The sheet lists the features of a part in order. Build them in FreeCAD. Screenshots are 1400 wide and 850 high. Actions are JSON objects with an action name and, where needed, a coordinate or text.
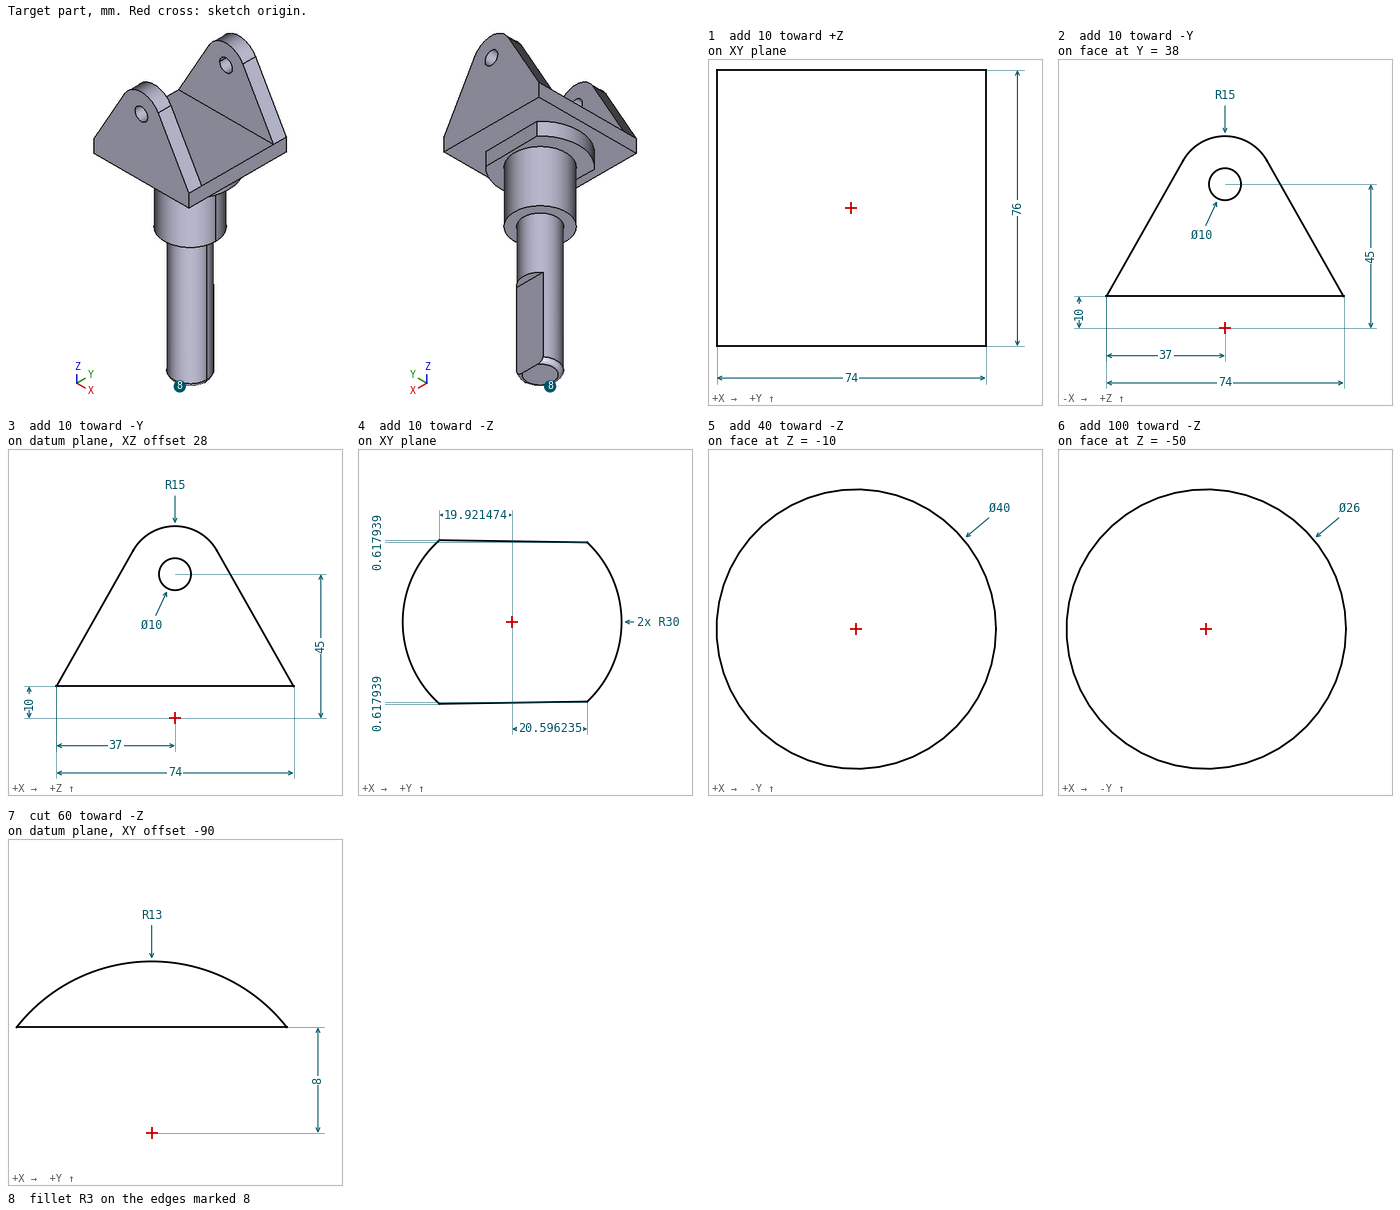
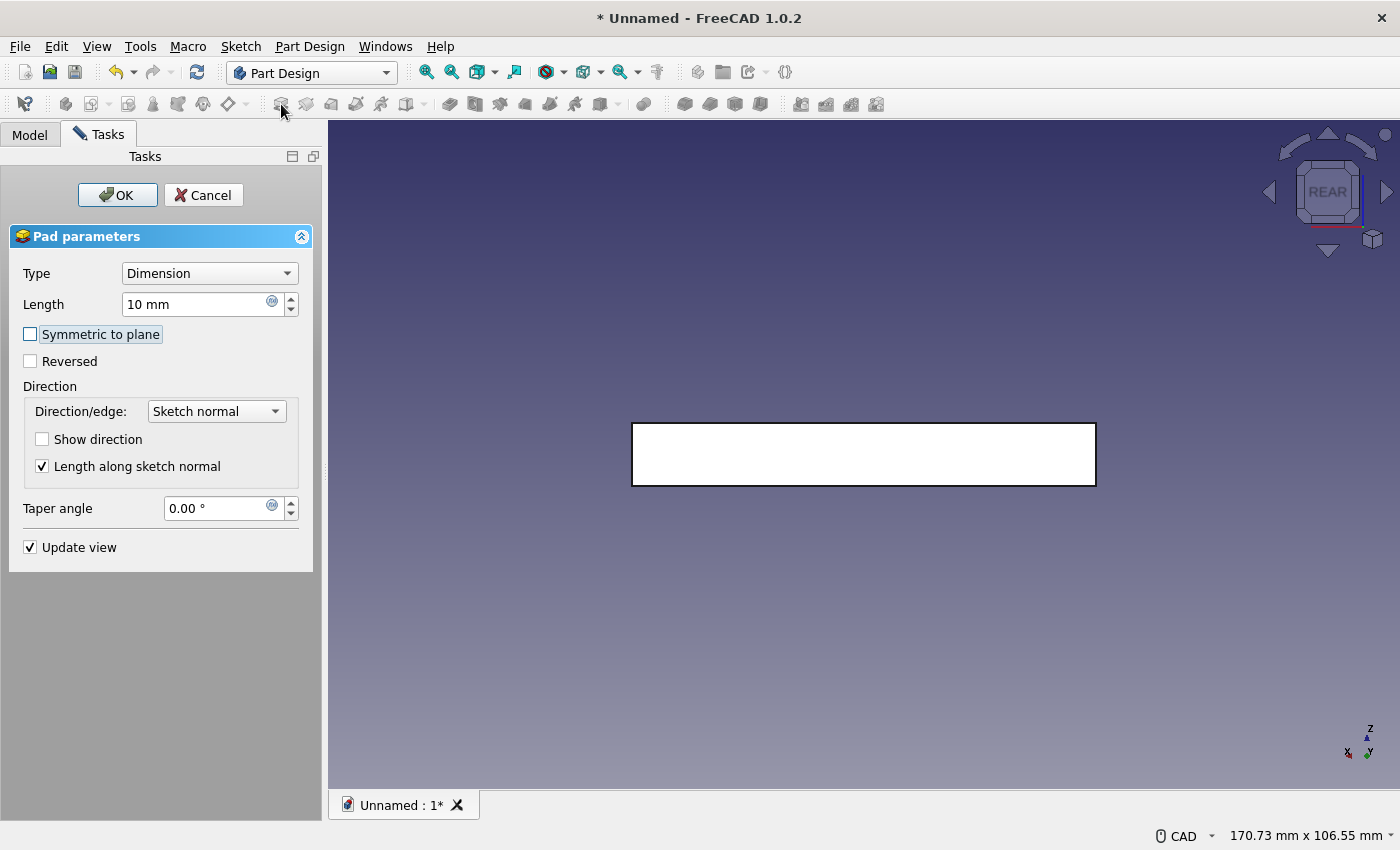
{"action": "left_click", "coordinate": [31, 361]}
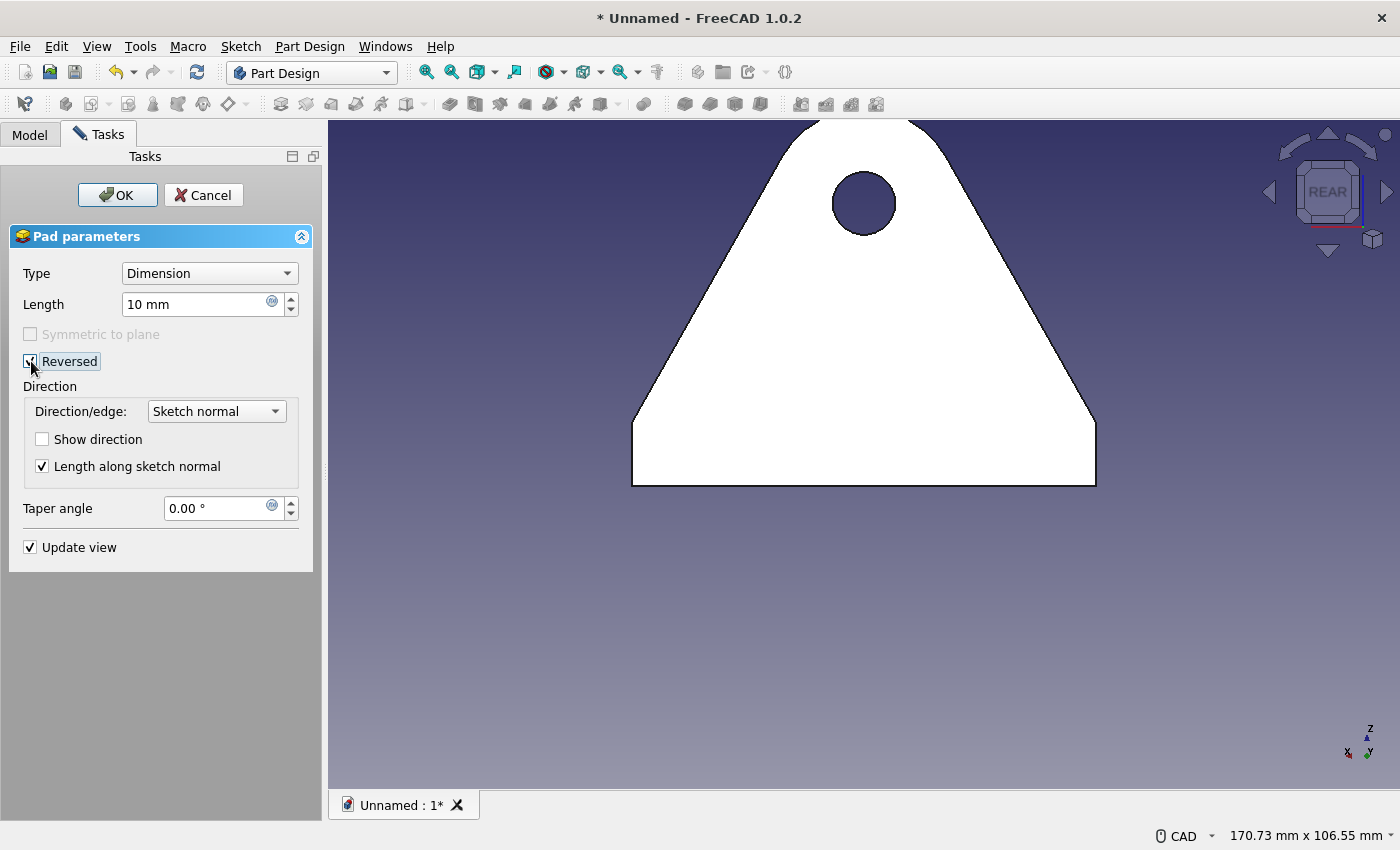
{"action": "left_click", "coordinate": [118, 195]}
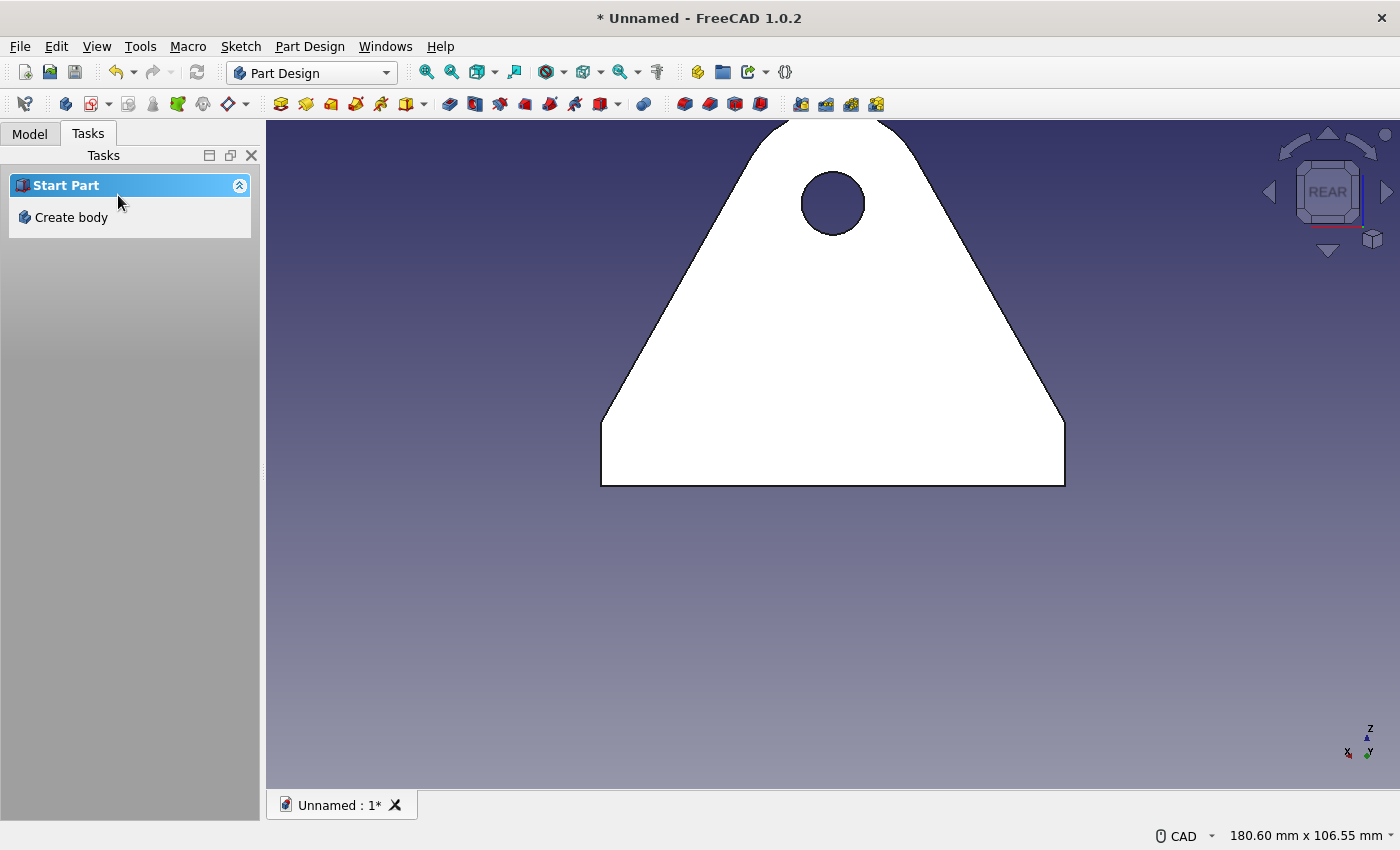
{"action": "left_click", "coordinate": [427, 72]}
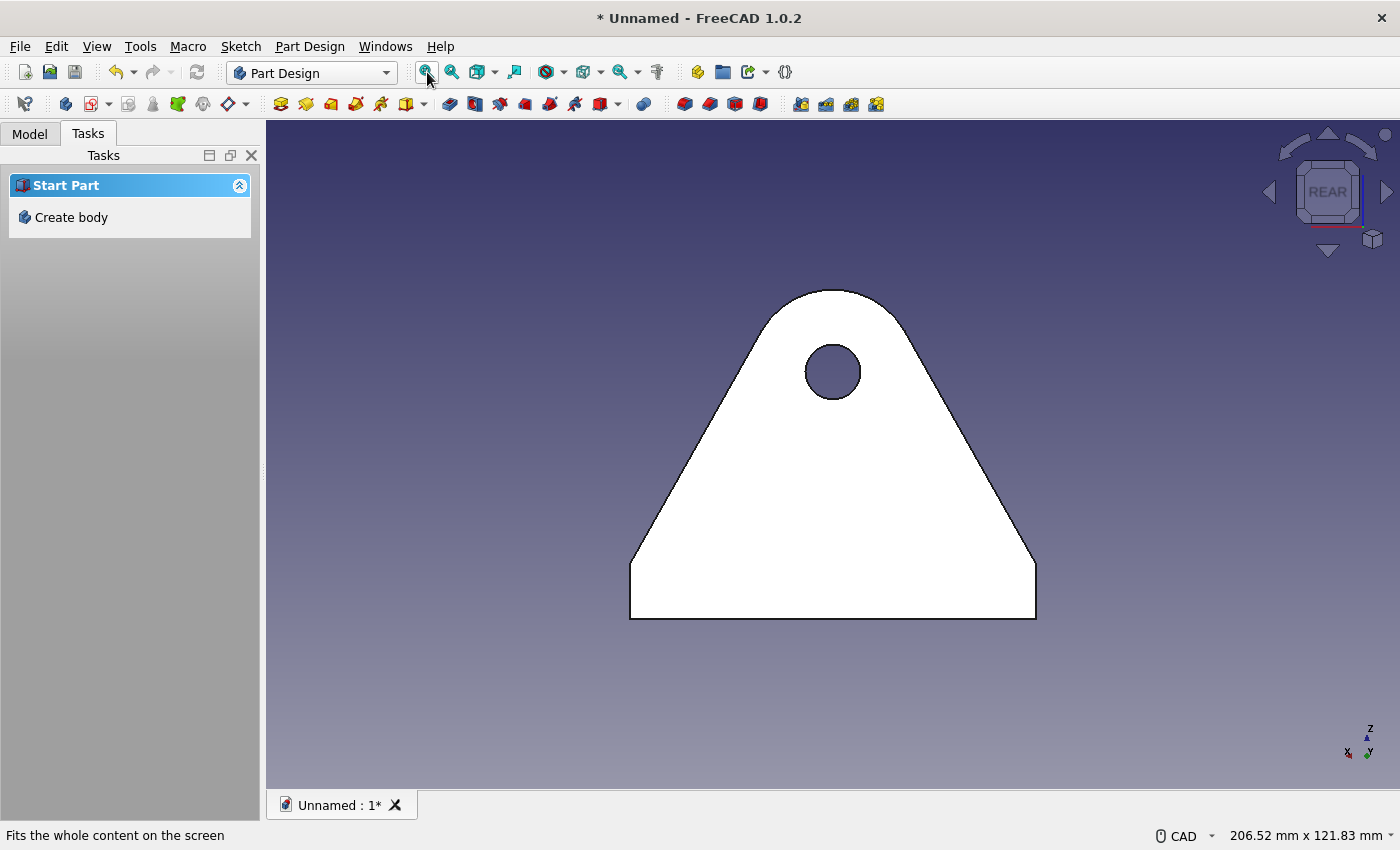
{"action": "left_click", "coordinate": [30, 134]}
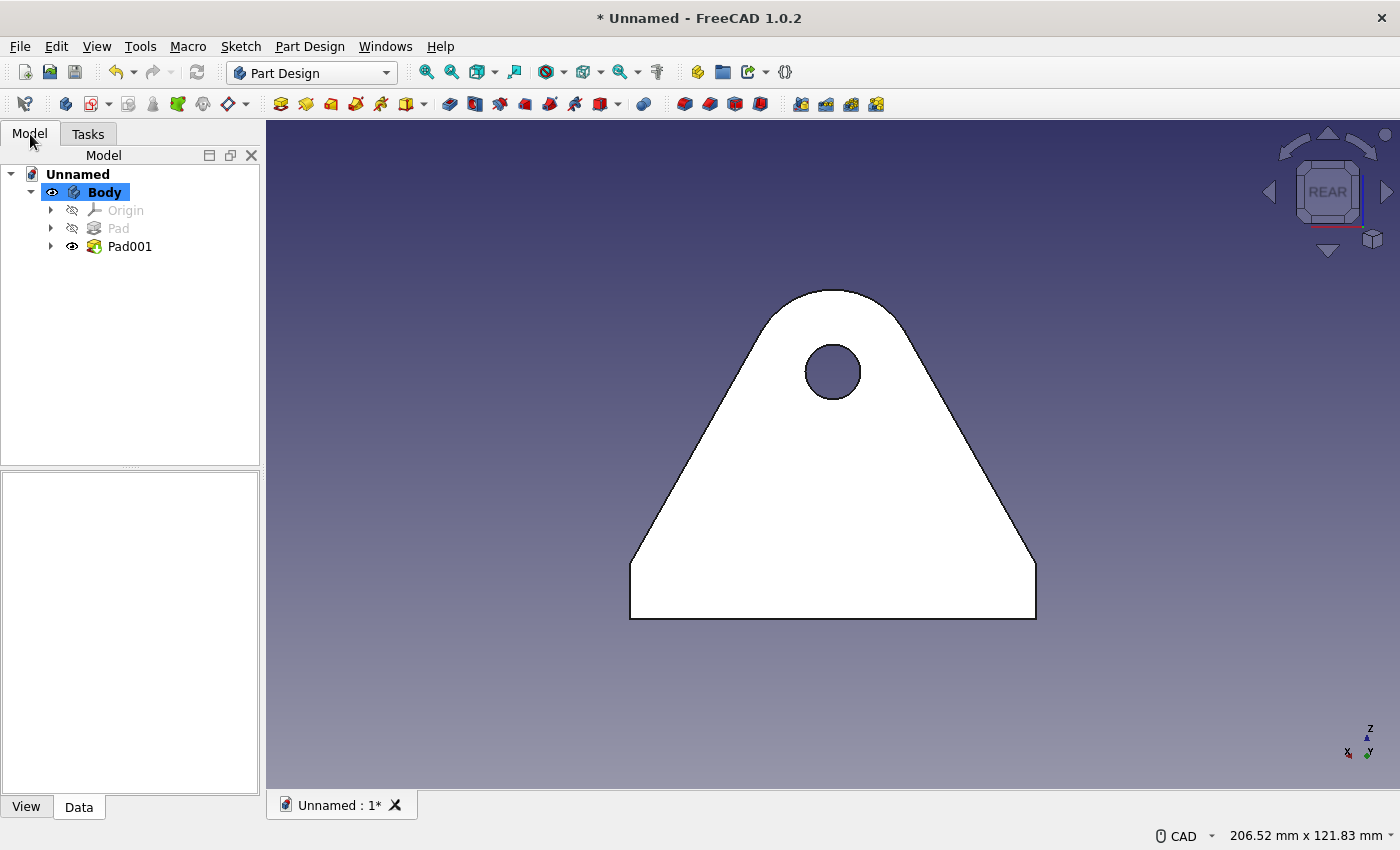
{"action": "left_click", "coordinate": [51, 210]}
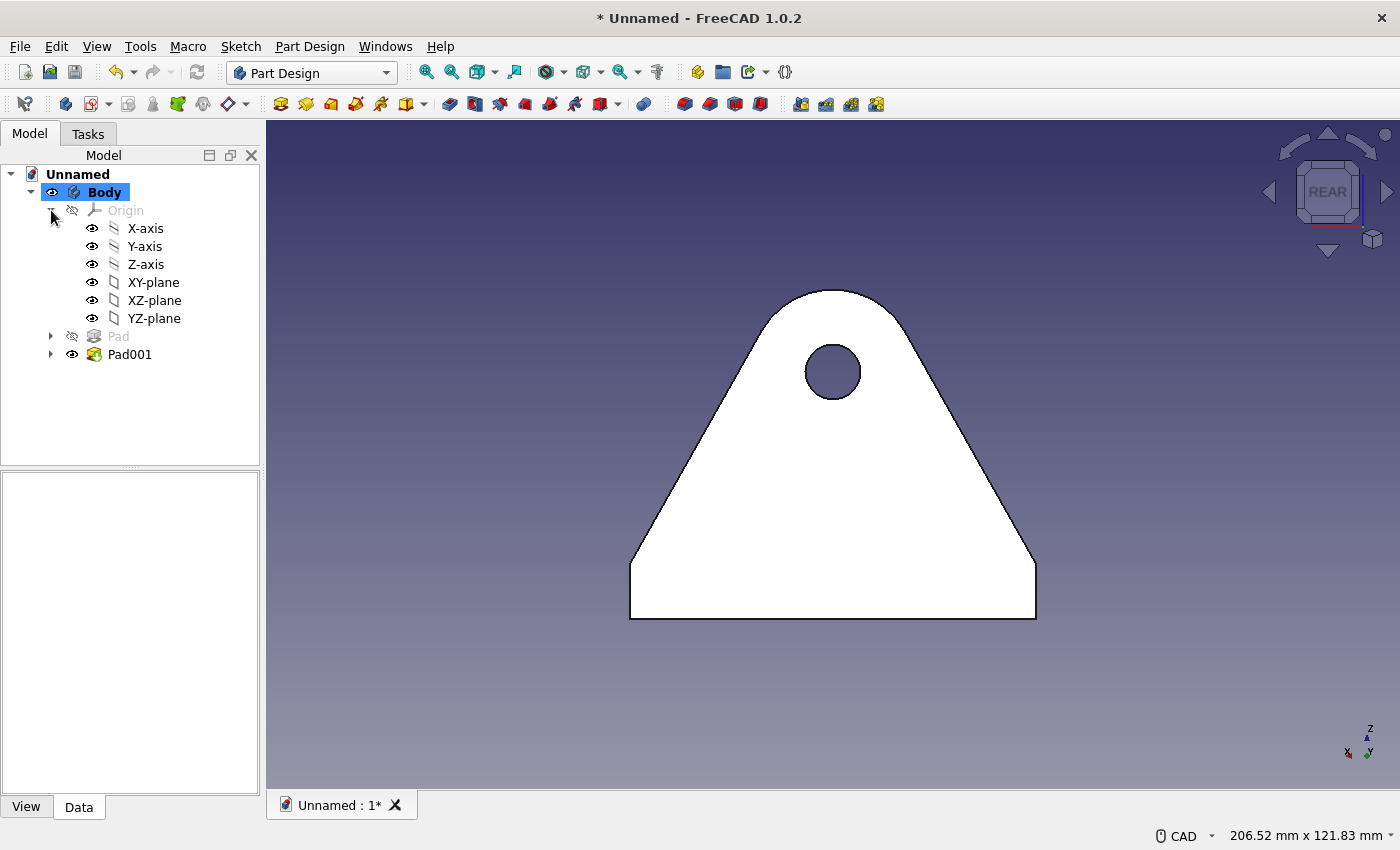
{"action": "left_click", "coordinate": [137, 300]}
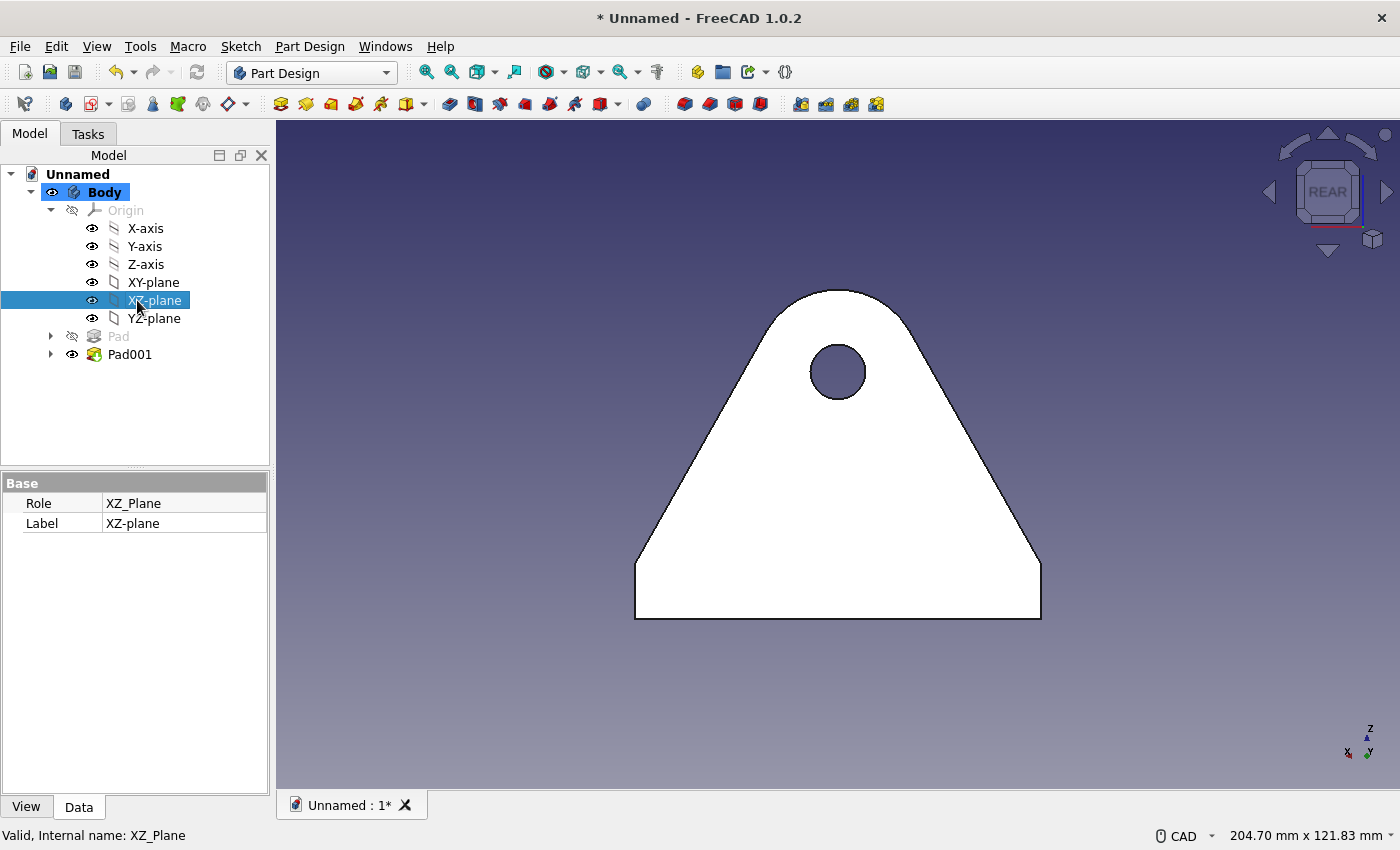
{"action": "left_click", "coordinate": [228, 104]}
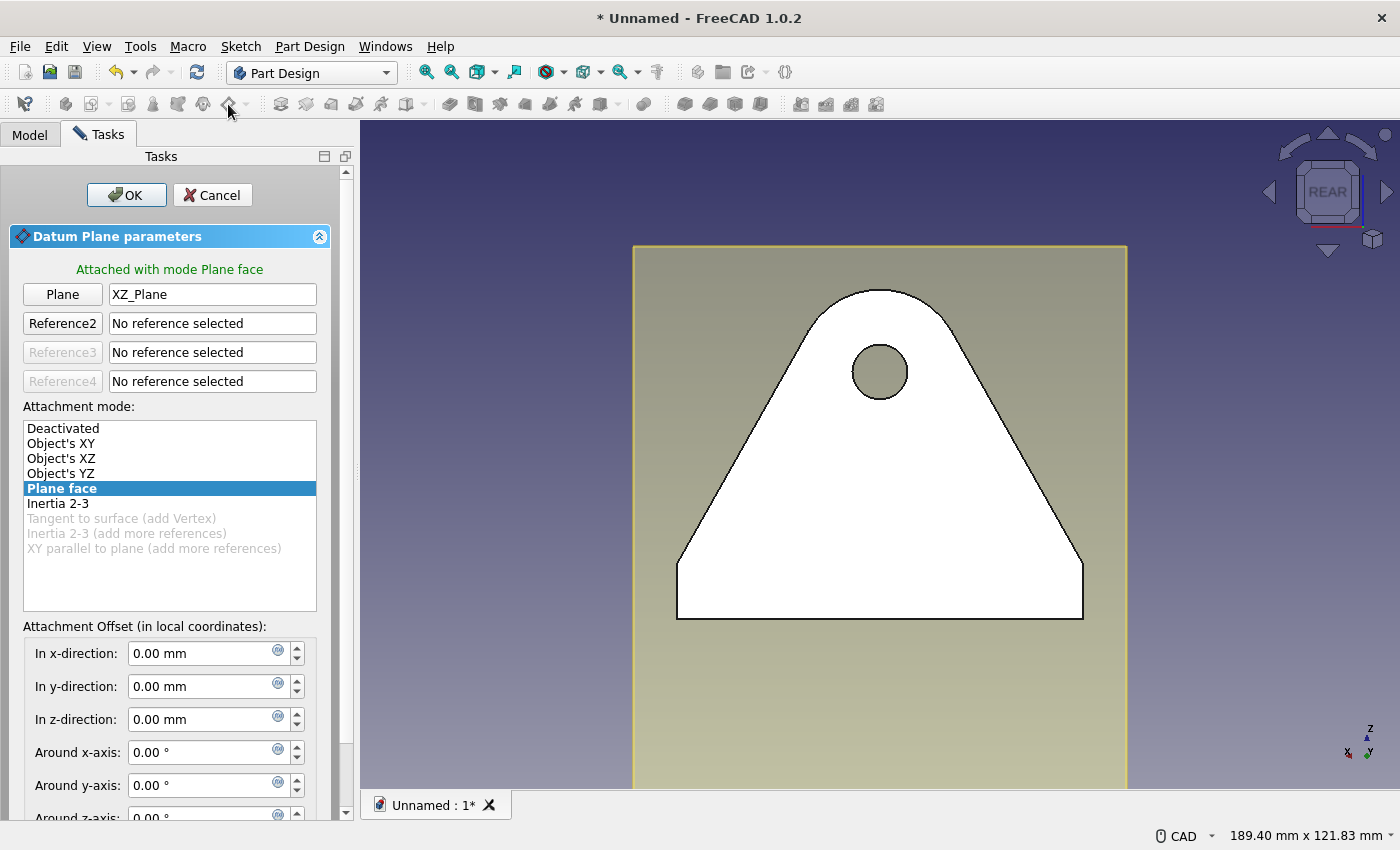
{"action": "triple_click", "coordinate": [210, 720]}